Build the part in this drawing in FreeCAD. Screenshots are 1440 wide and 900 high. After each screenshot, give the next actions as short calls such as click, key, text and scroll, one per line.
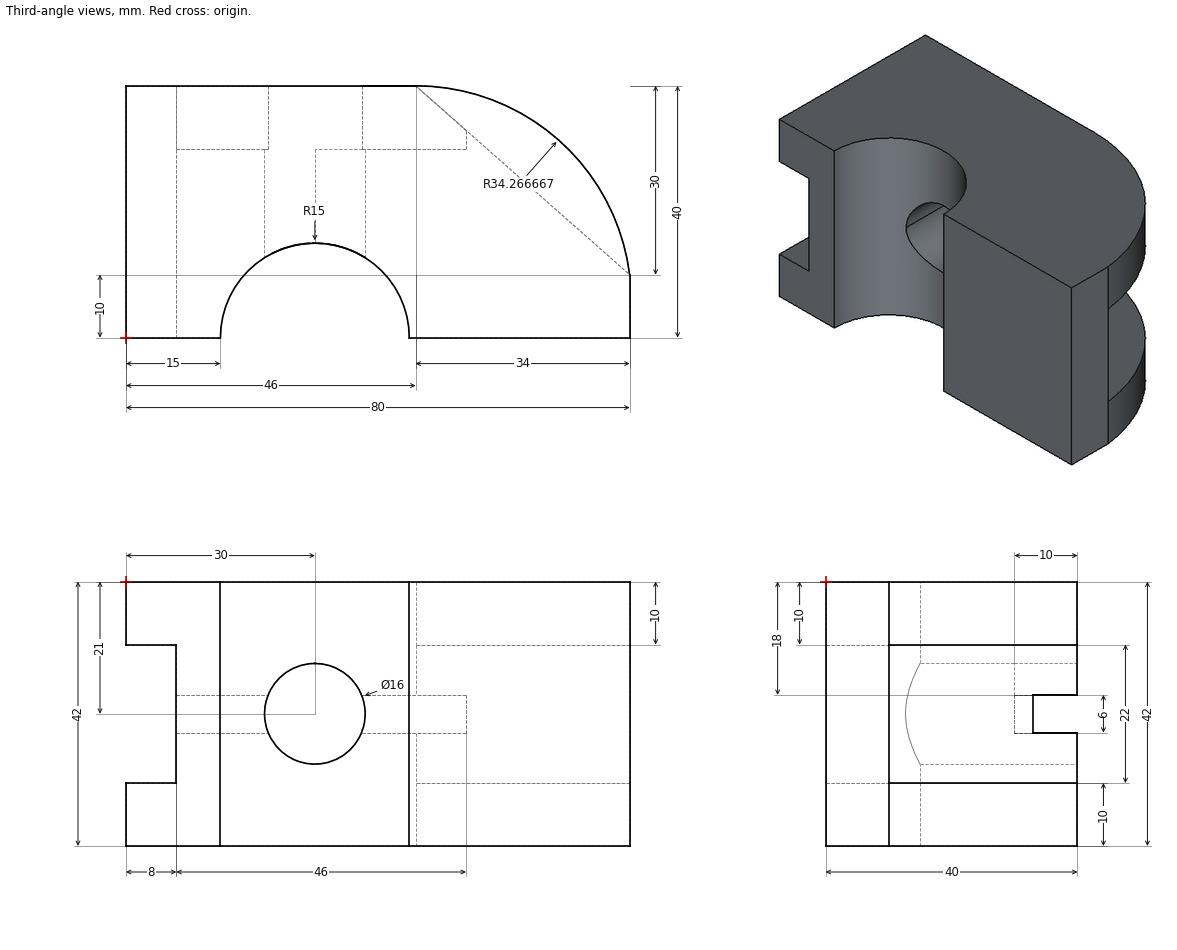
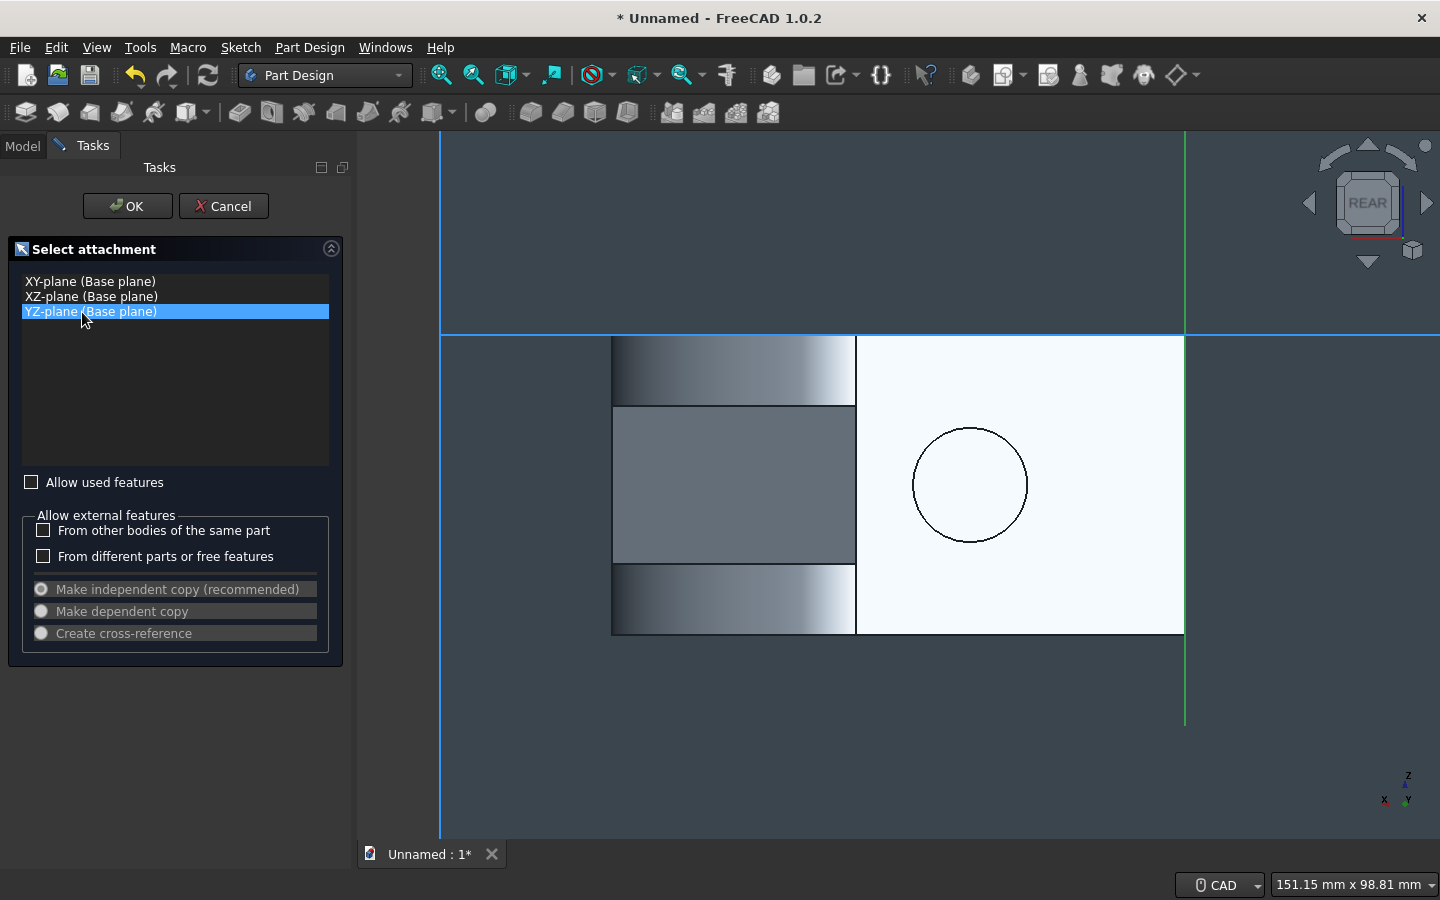
click(128, 206)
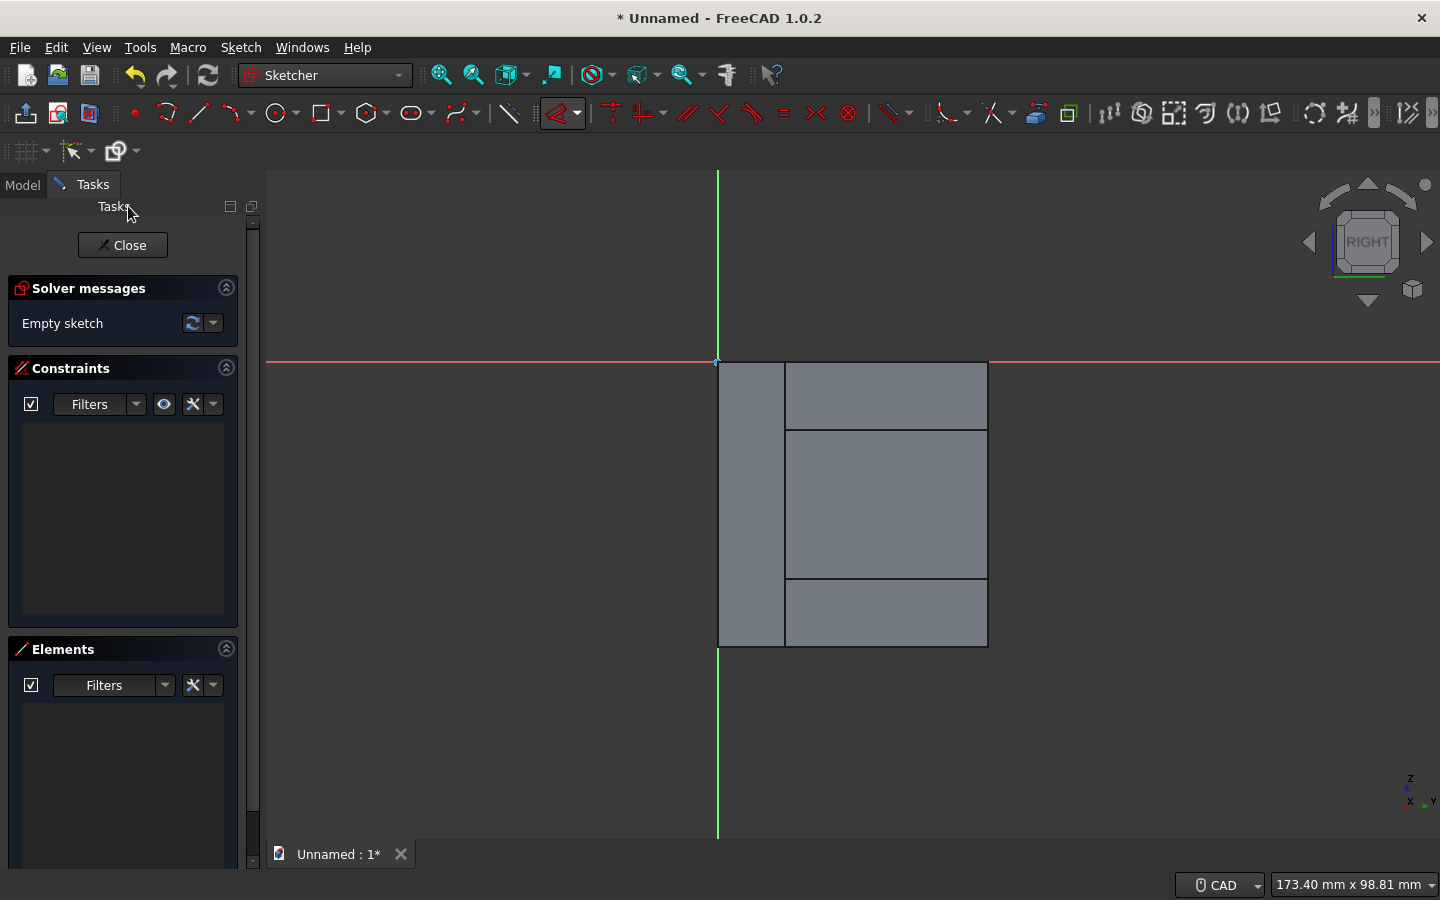
click(90, 114)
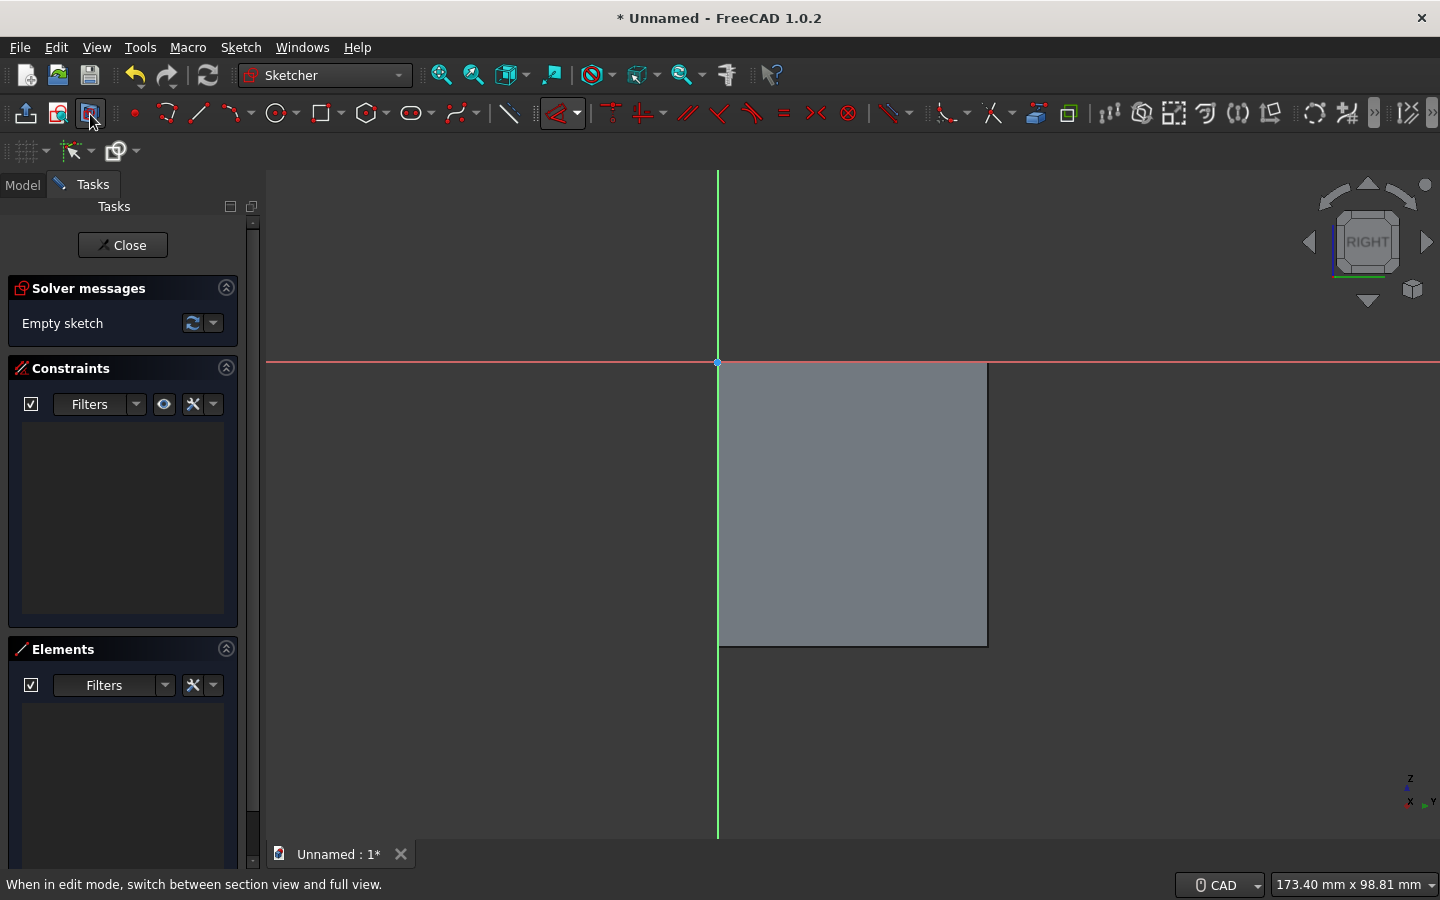
scroll(936, 429, up, 3)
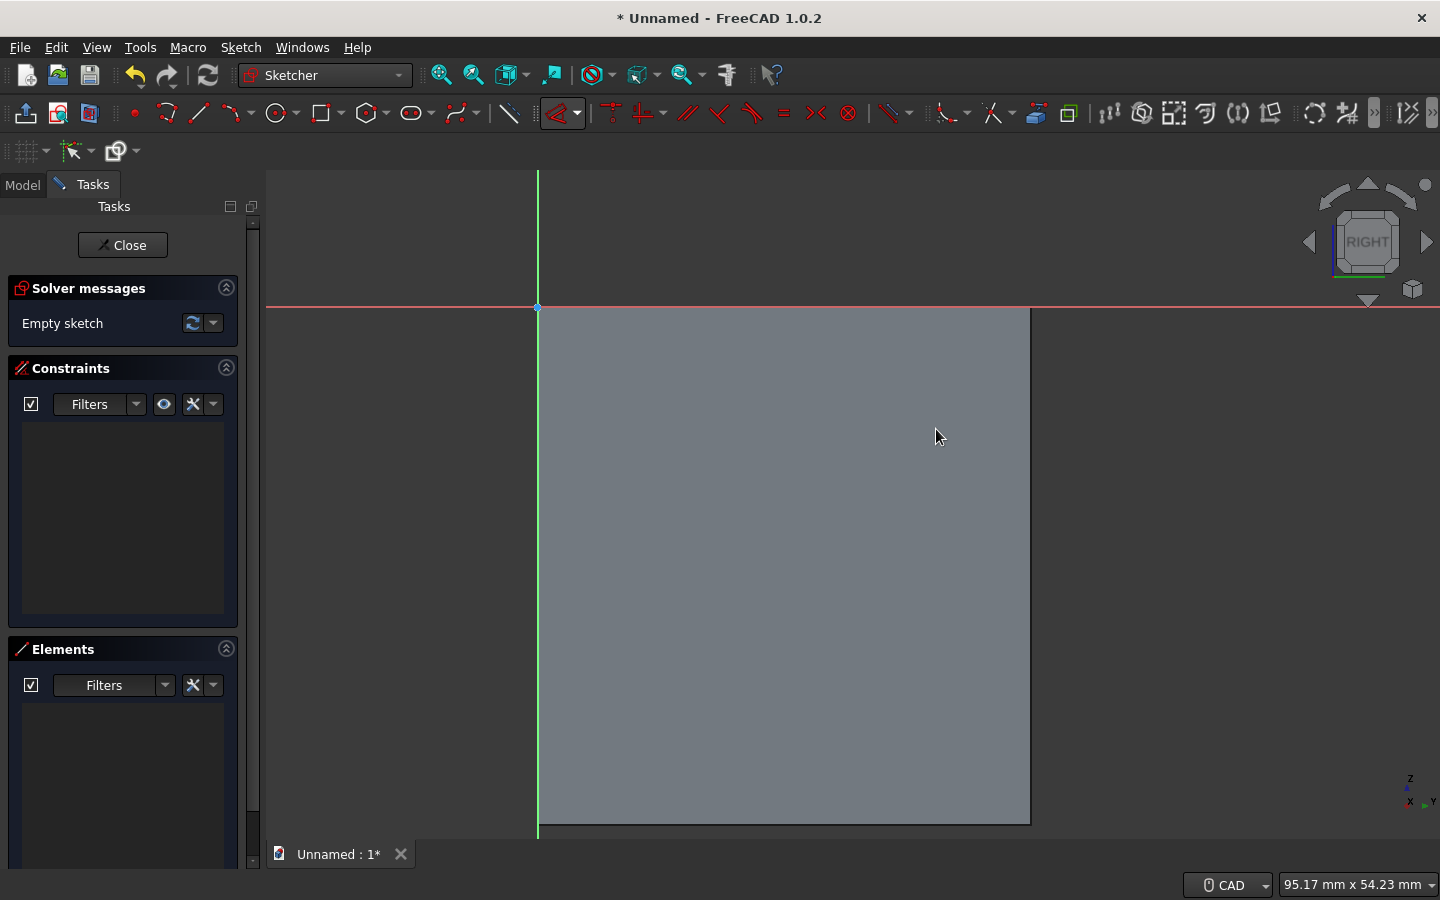
click(322, 114)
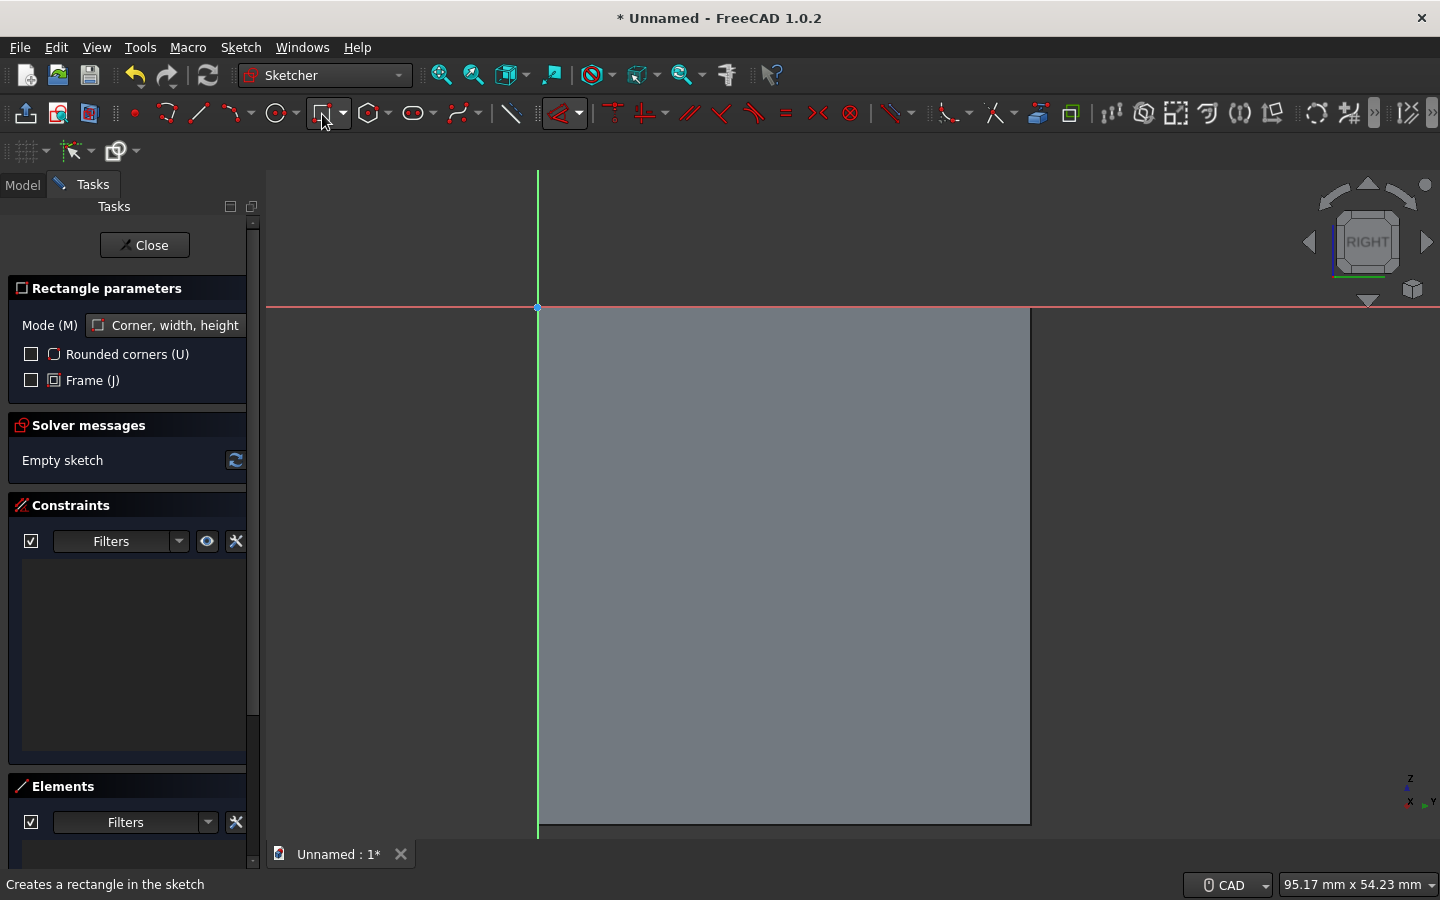
click(538, 431)
move(1031, 702)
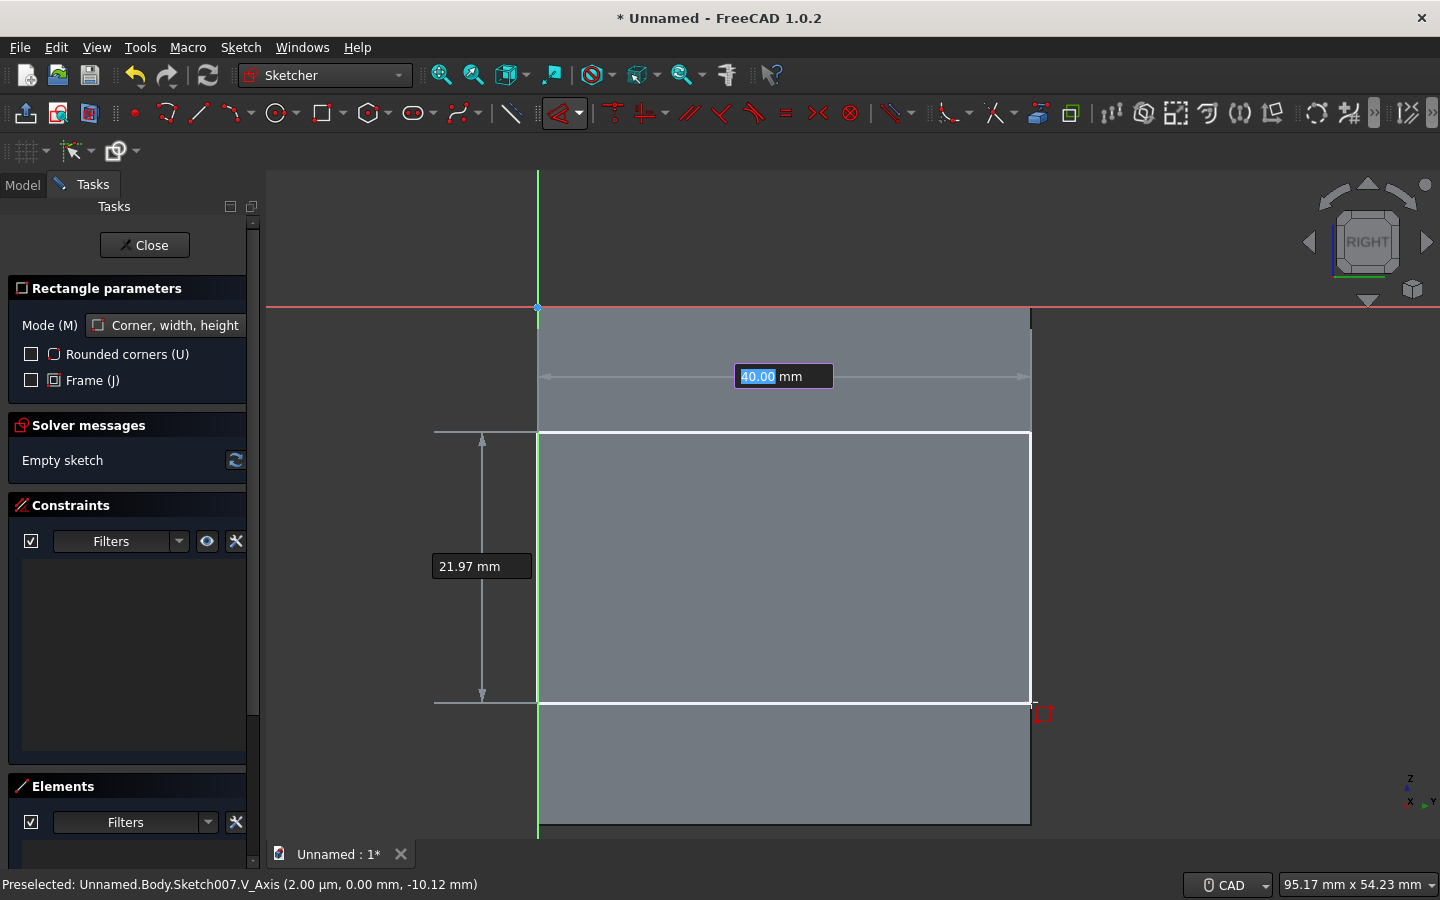
text(40)
key(Tab)
text(22)
key(Return)
key(Escape)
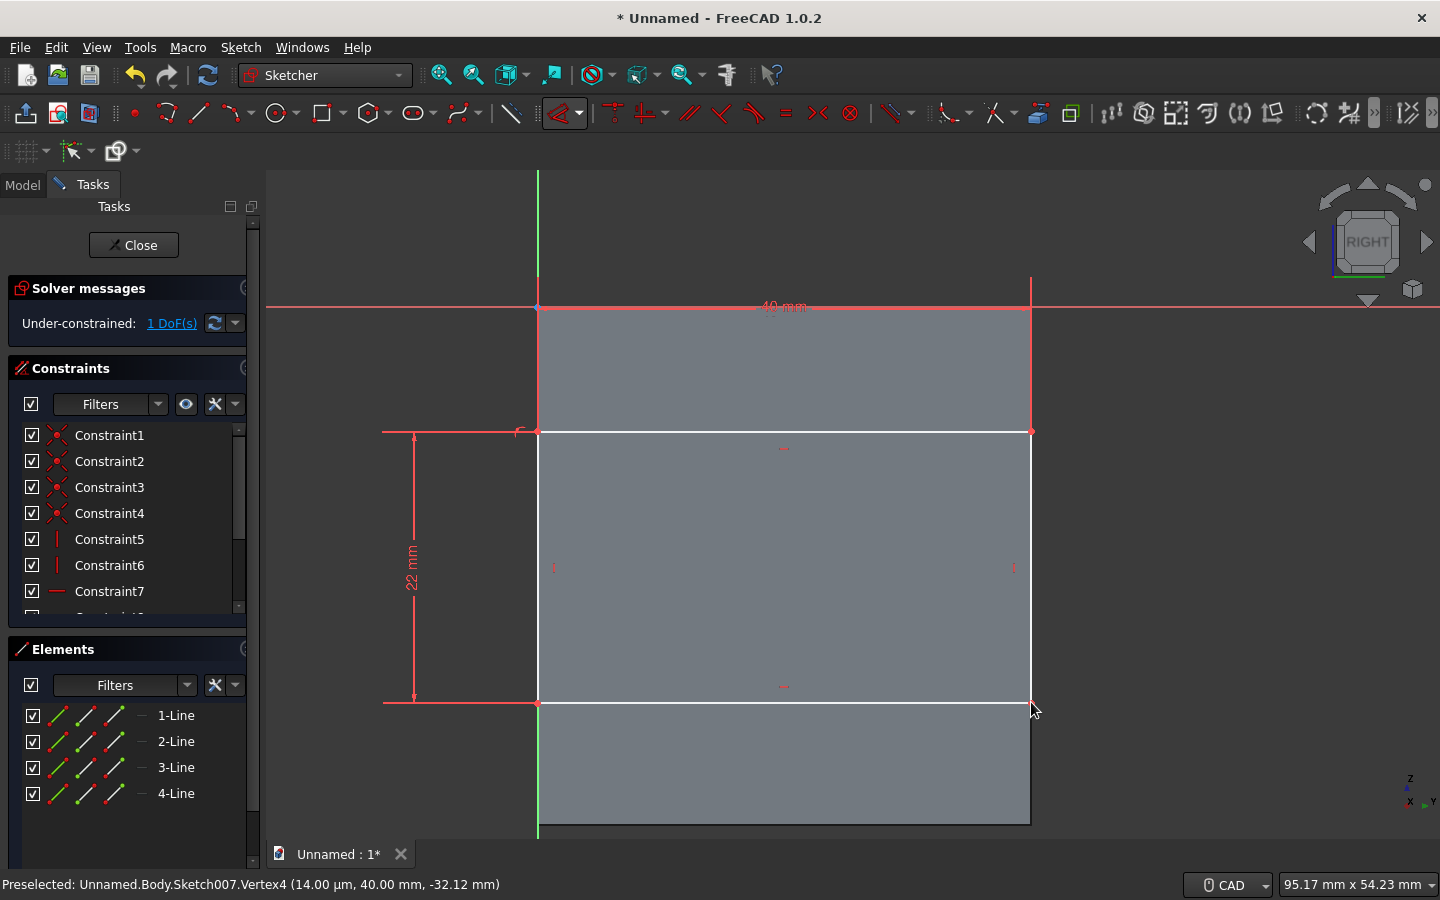
click(538, 432)